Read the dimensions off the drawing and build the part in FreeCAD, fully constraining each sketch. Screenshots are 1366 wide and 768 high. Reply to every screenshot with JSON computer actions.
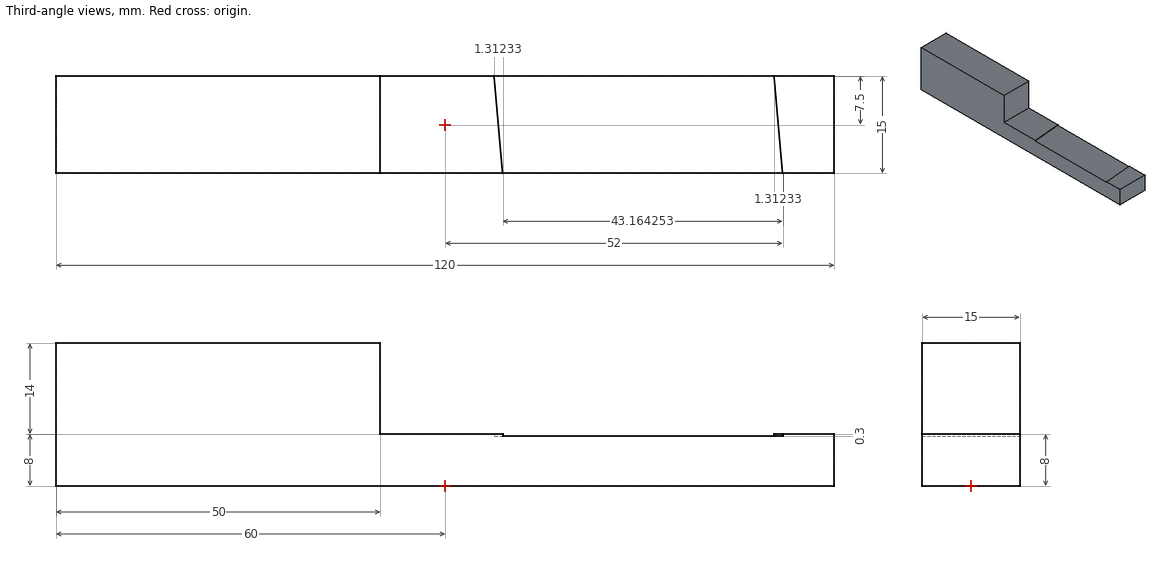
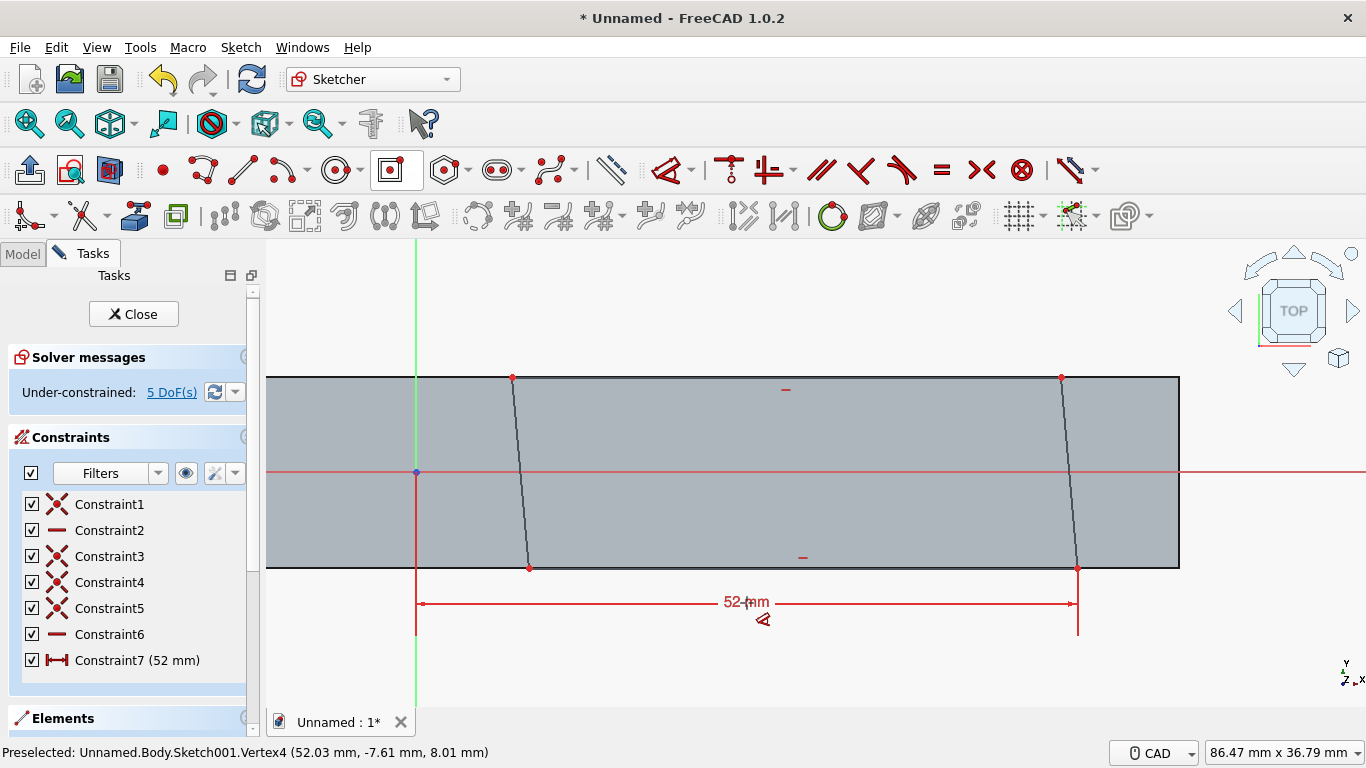
{"action": "left_click", "coordinate": [517, 435]}
{"action": "left_click", "coordinate": [478, 430]}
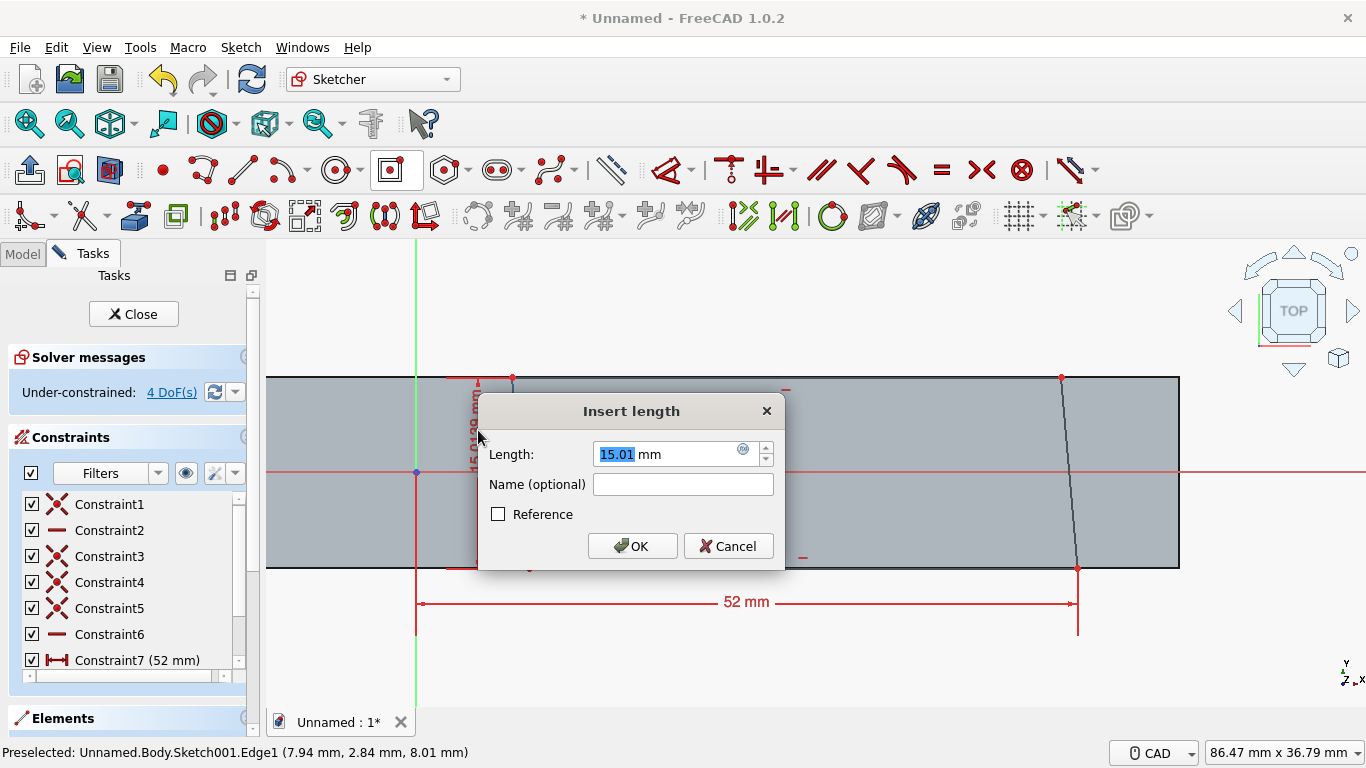
{"action": "type", "text": "15"}
{"action": "key", "text": "Return"}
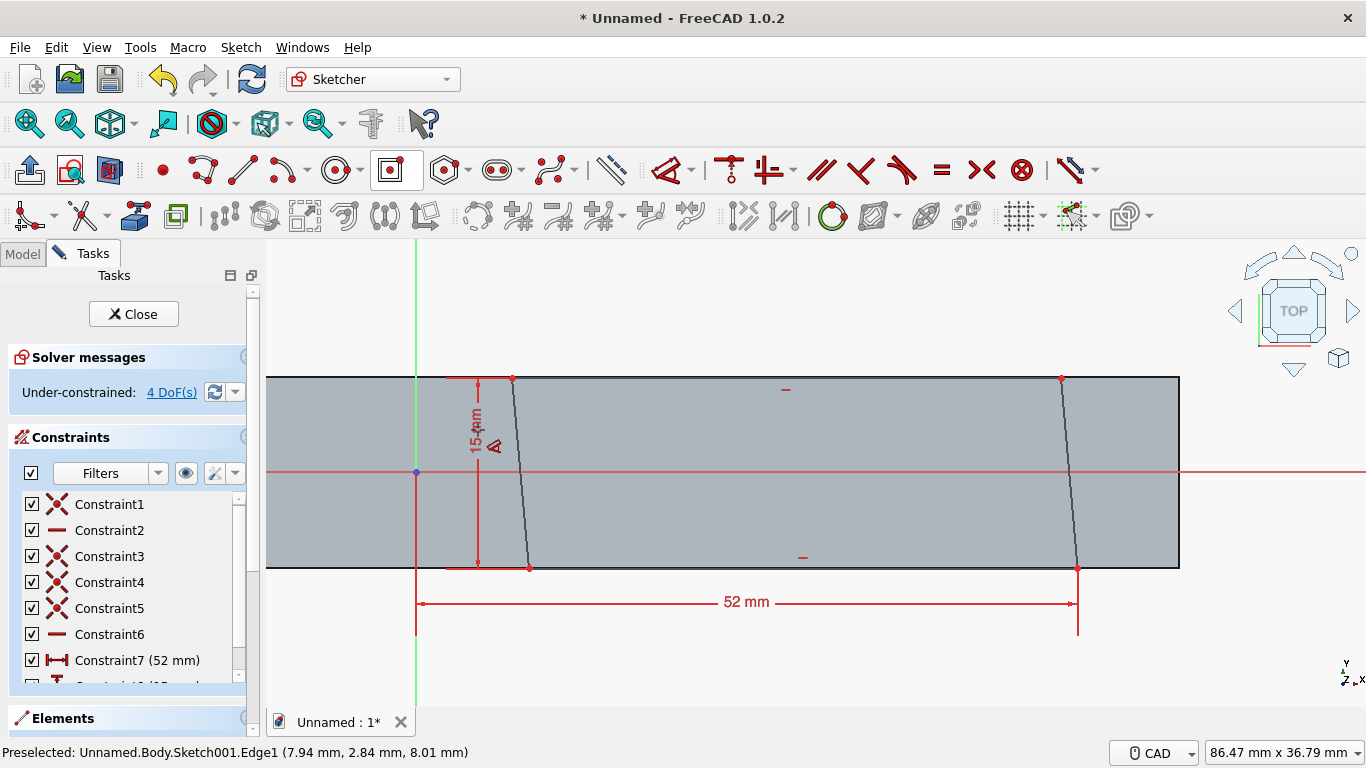
{"action": "left_click", "coordinate": [512, 378]}
{"action": "left_click", "coordinate": [382, 425]}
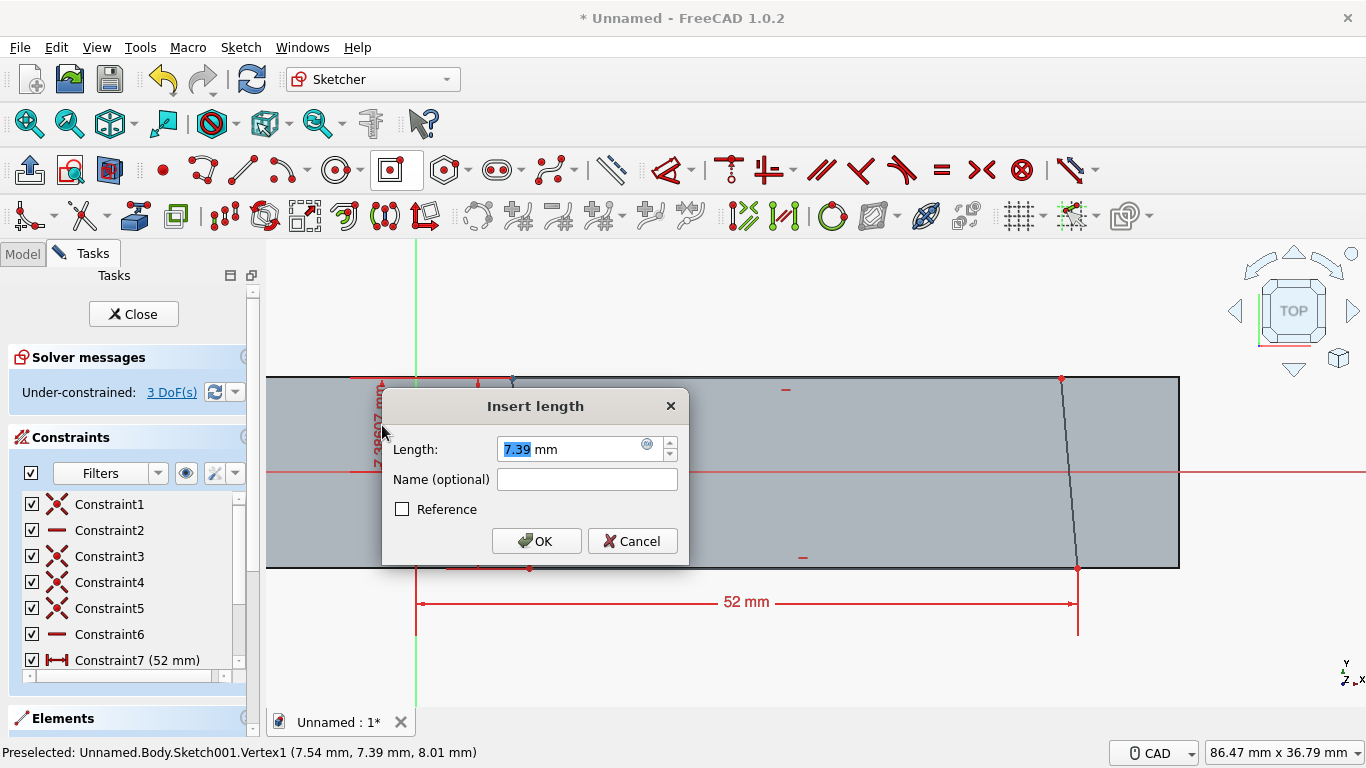
{"action": "type", "text": "7.5"}
{"action": "key", "text": "Return"}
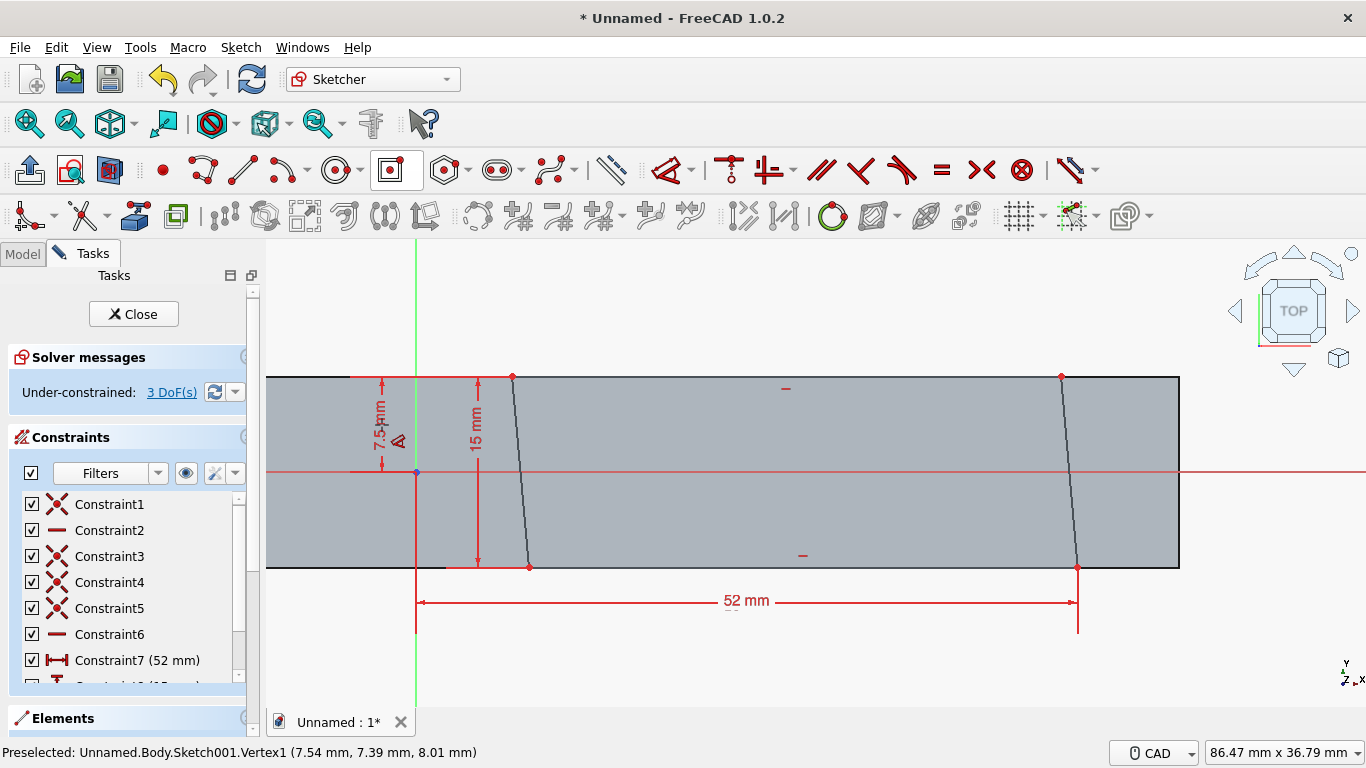
{"action": "scroll", "coordinate": [517, 434], "scroll_direction": "up", "scroll_amount": 5}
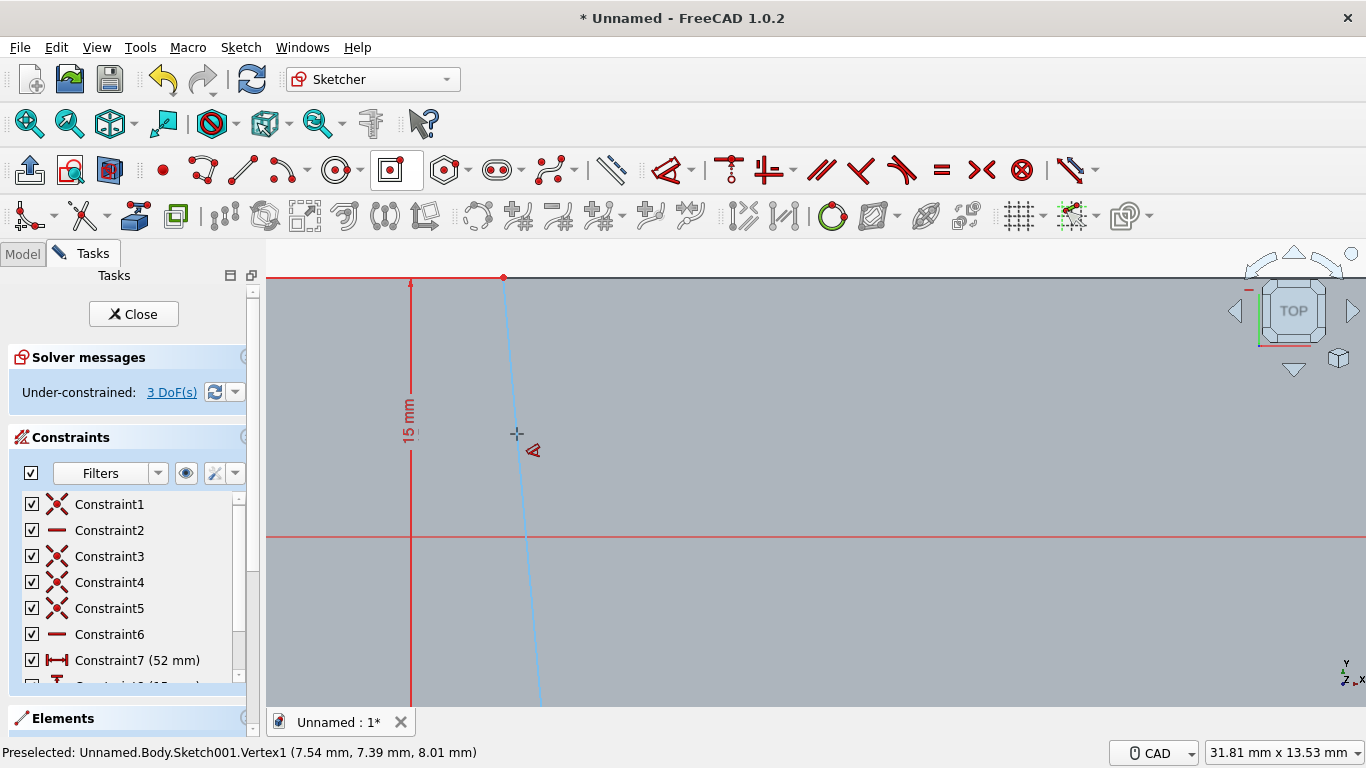
{"action": "left_click", "coordinate": [517, 433]}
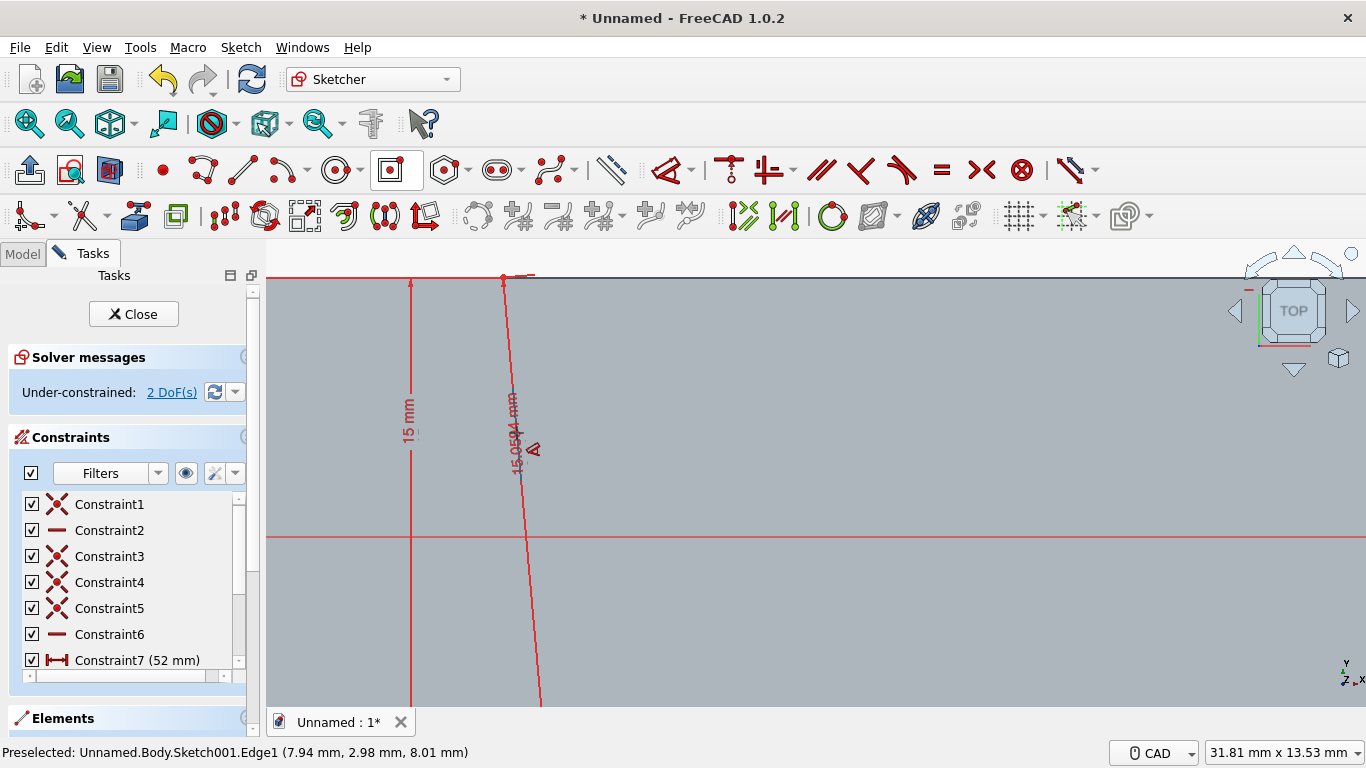
{"action": "key", "text": "Escape"}
{"action": "key", "text": "Escape"}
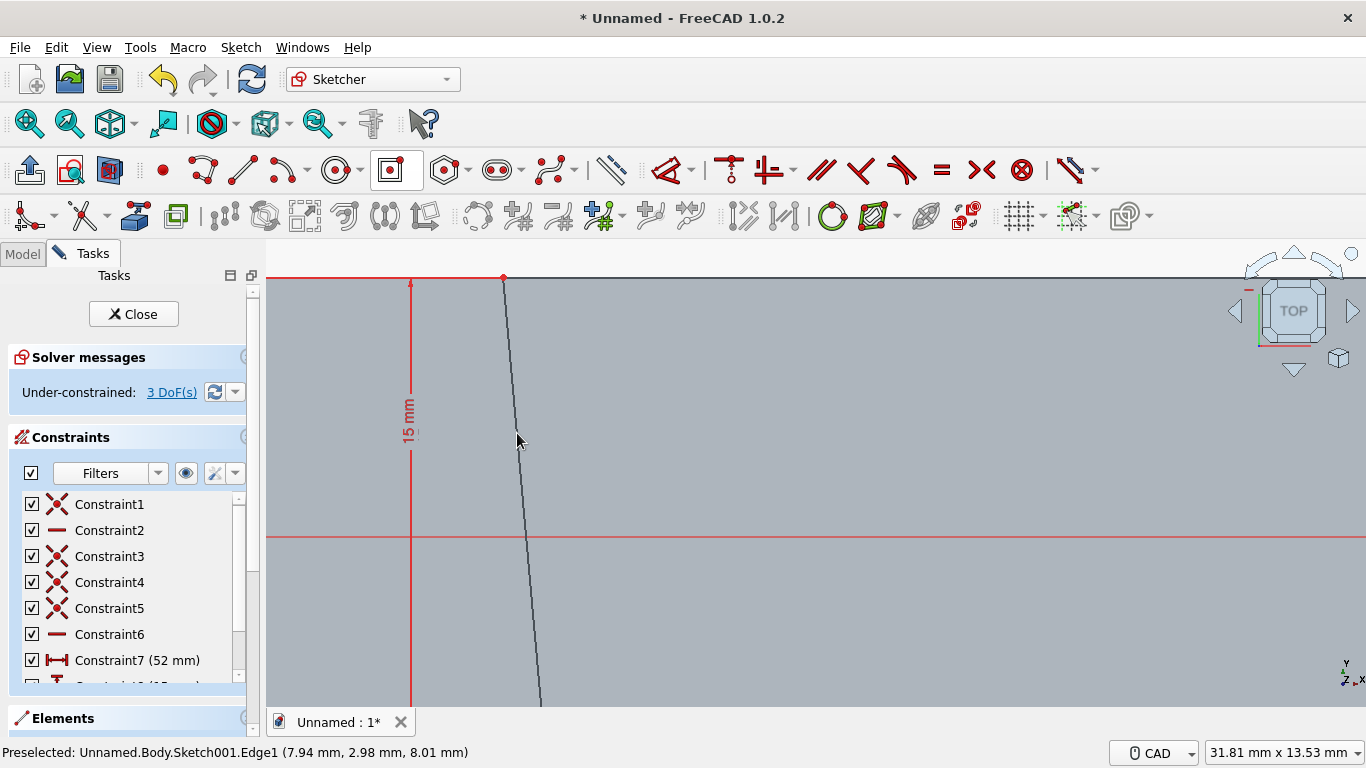
{"action": "left_click", "coordinate": [517, 433]}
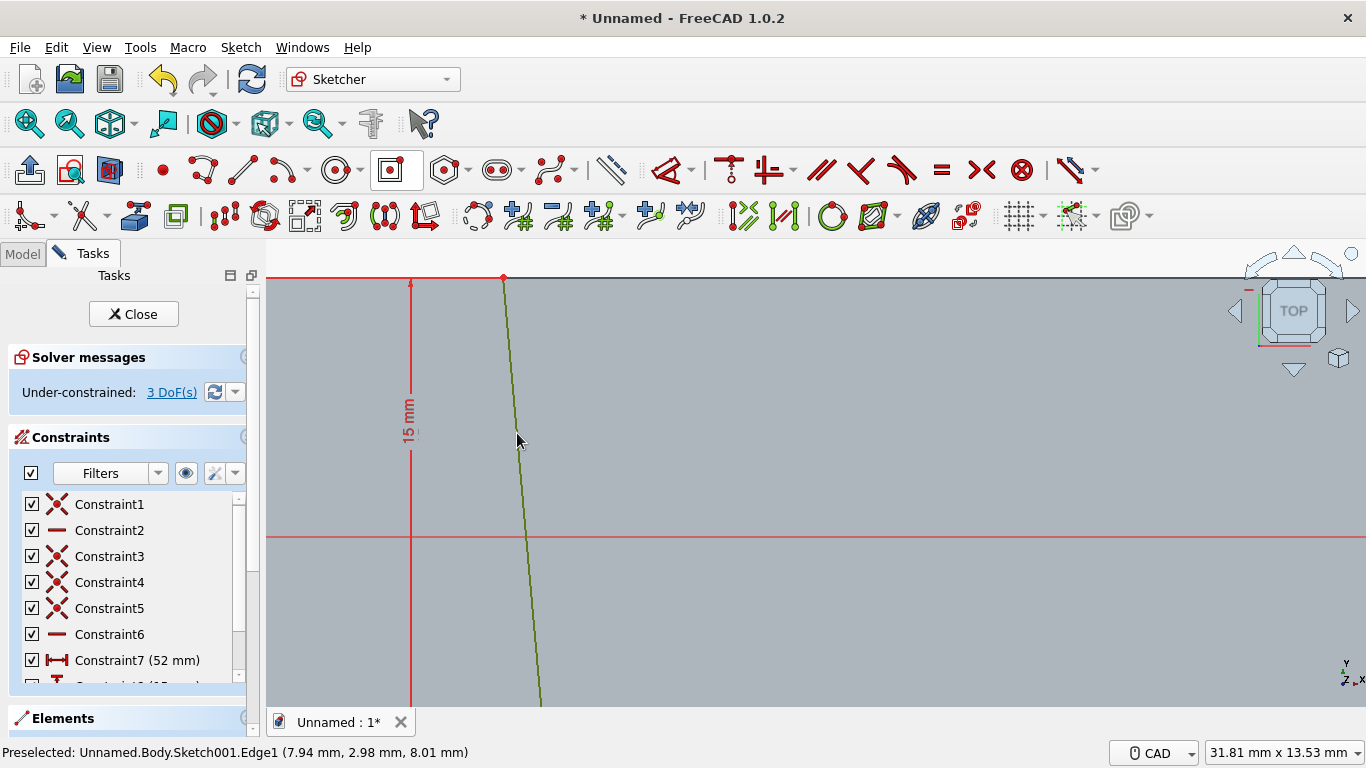
{"action": "left_click", "coordinate": [694, 170]}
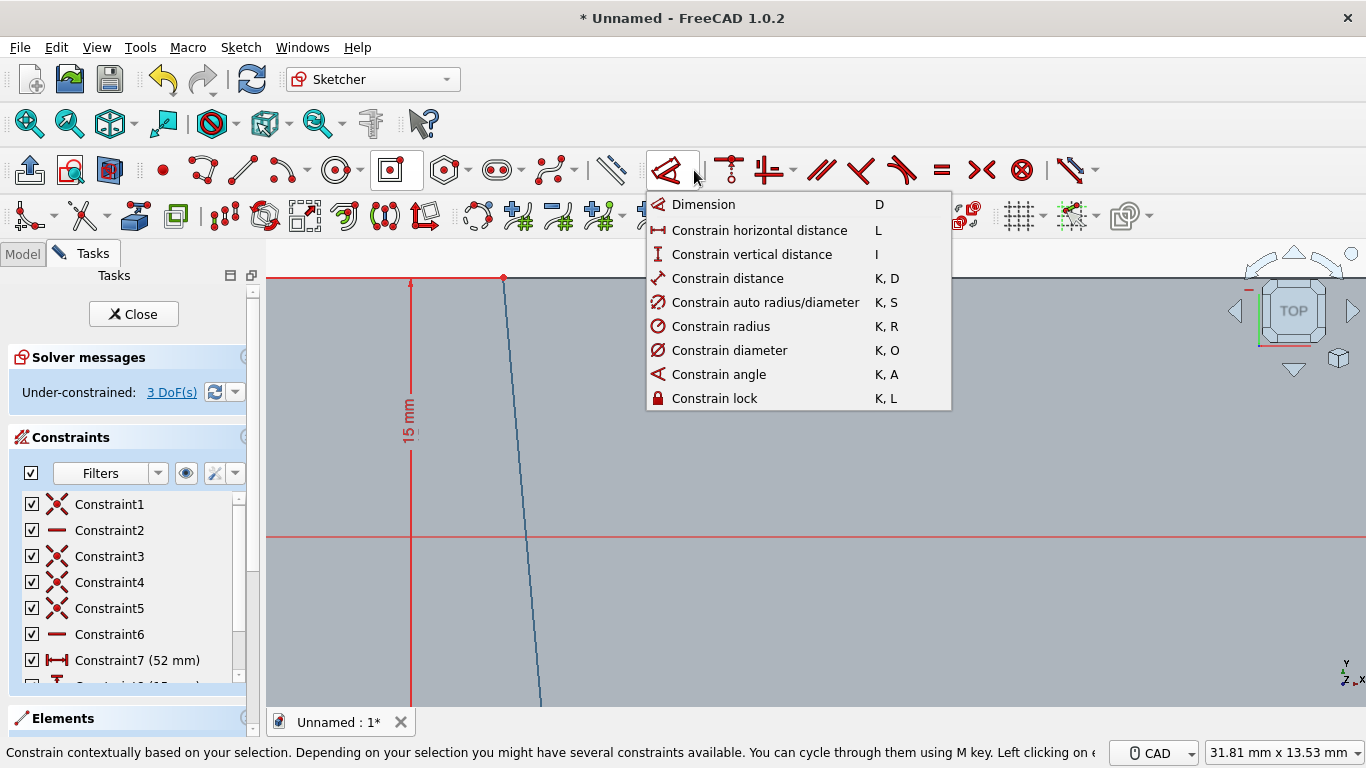
{"action": "left_click", "coordinate": [799, 230]}